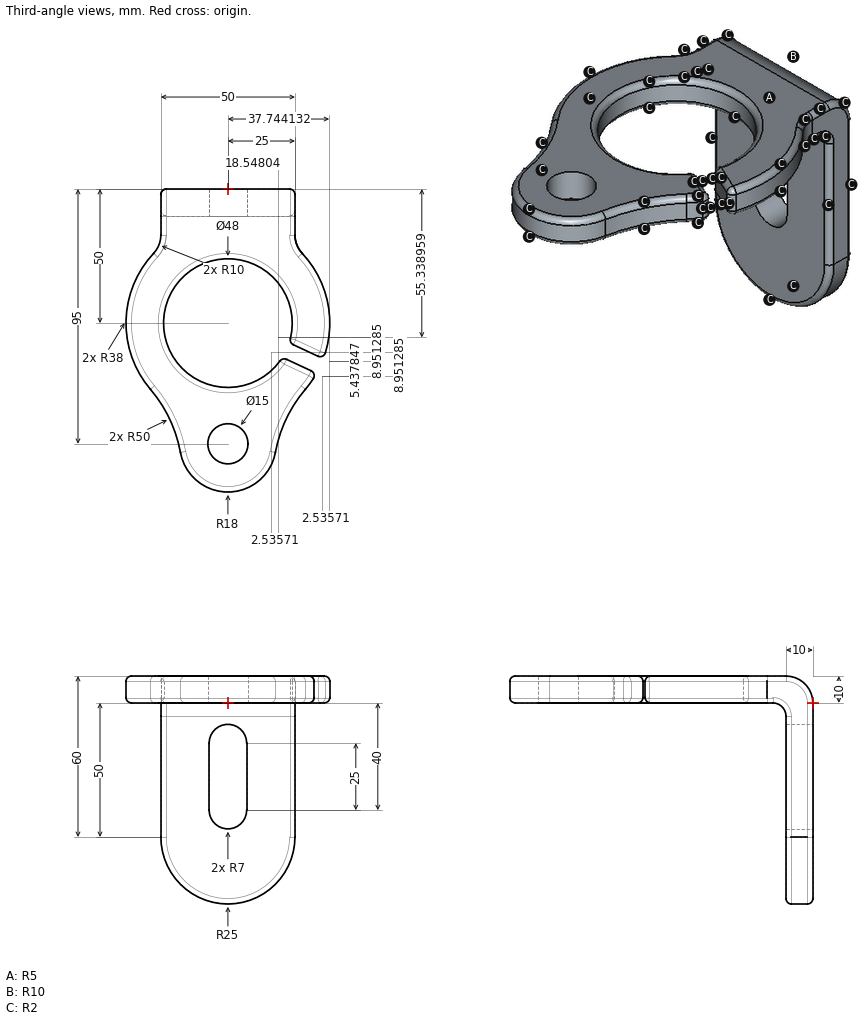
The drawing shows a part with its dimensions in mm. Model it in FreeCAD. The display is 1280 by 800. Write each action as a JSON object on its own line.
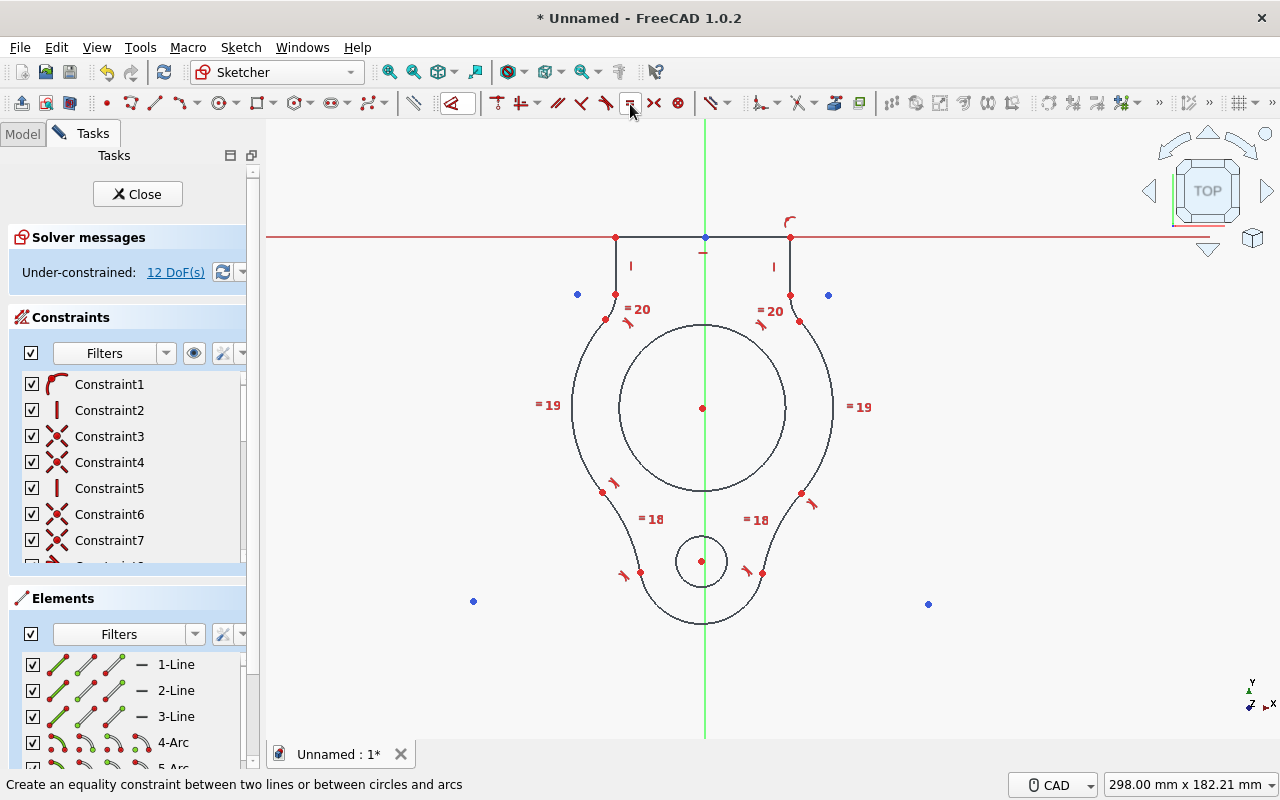
{"action": "left_click", "coordinate": [702, 408]}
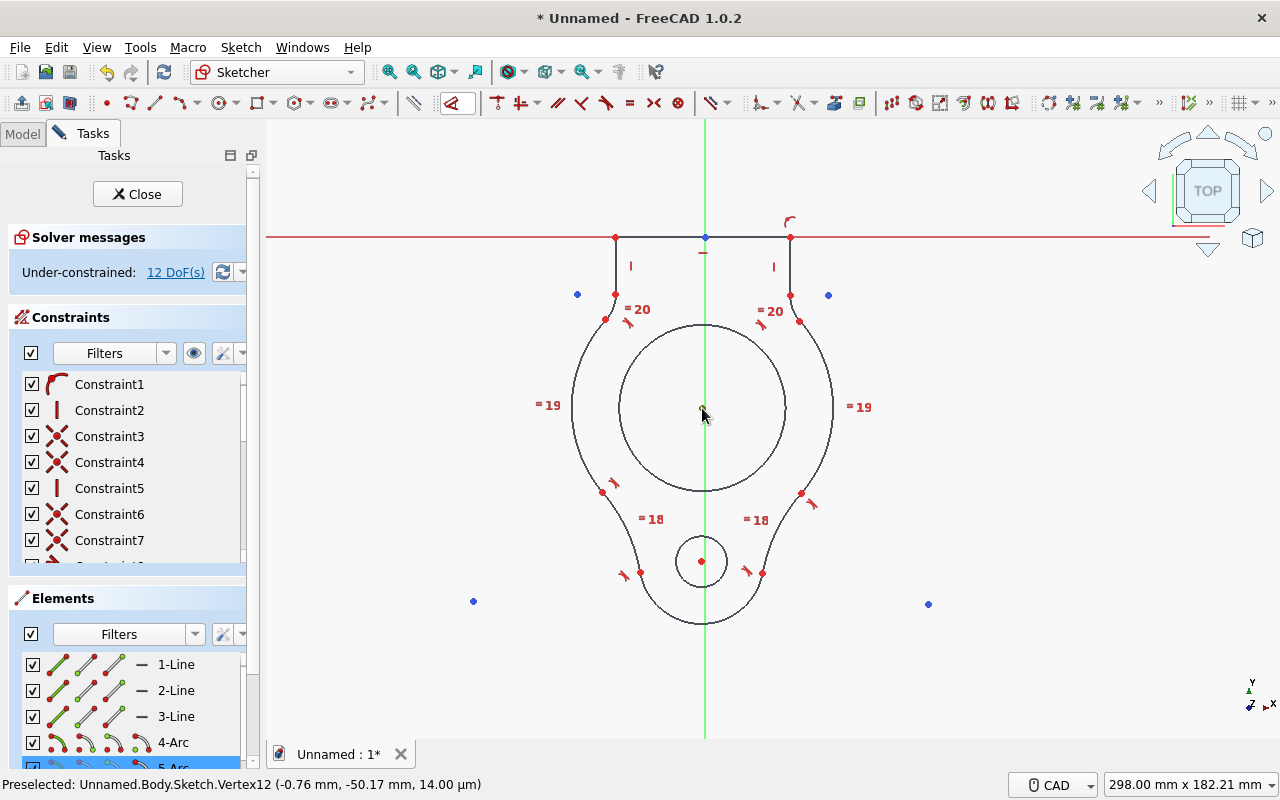
{"action": "left_click", "coordinate": [705, 671]}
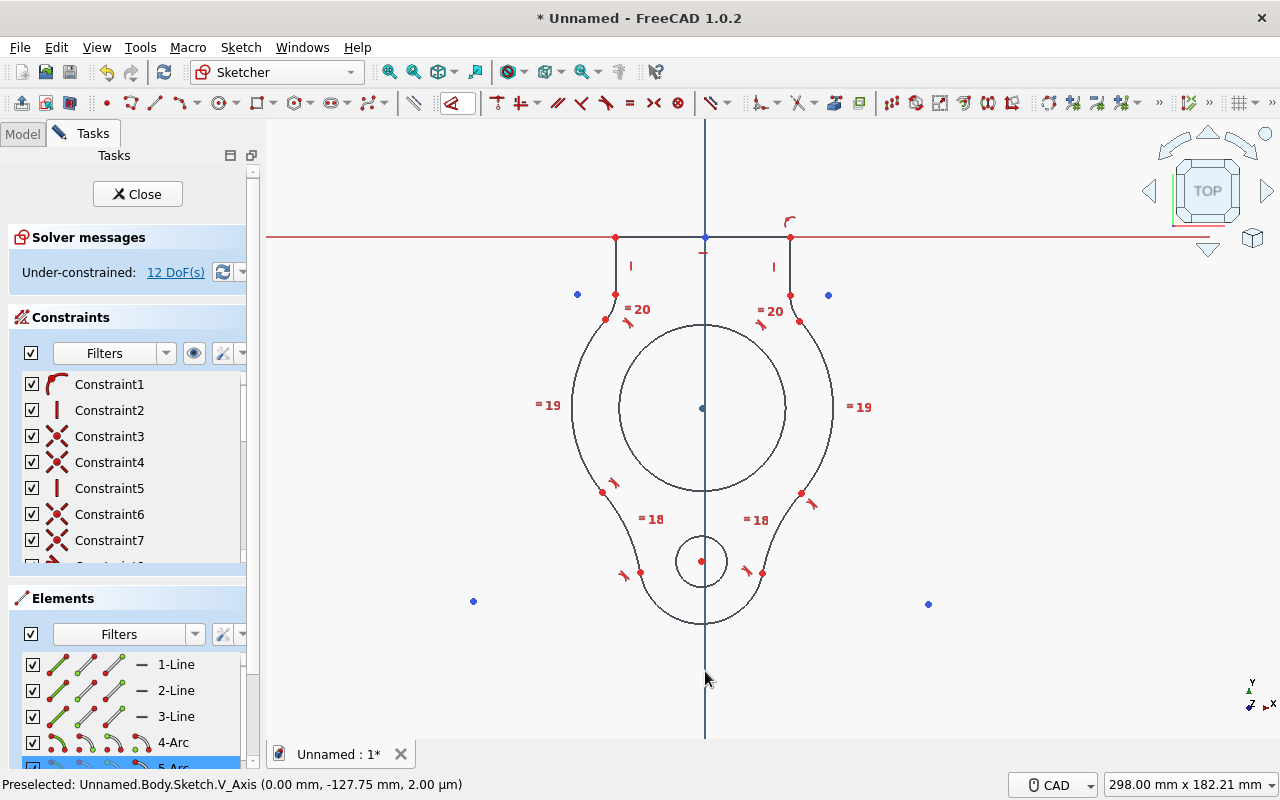
{"action": "left_click", "coordinate": [498, 104]}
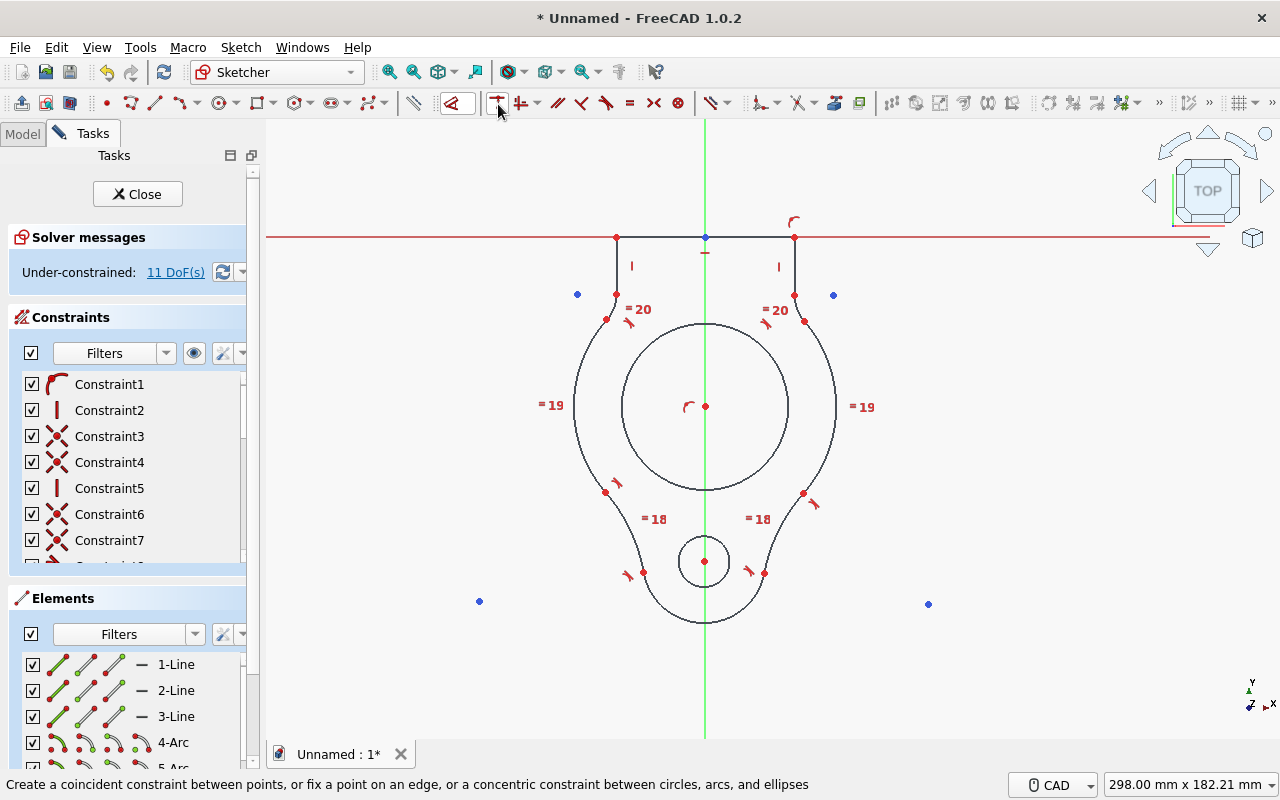
{"action": "left_click", "coordinate": [704, 562]}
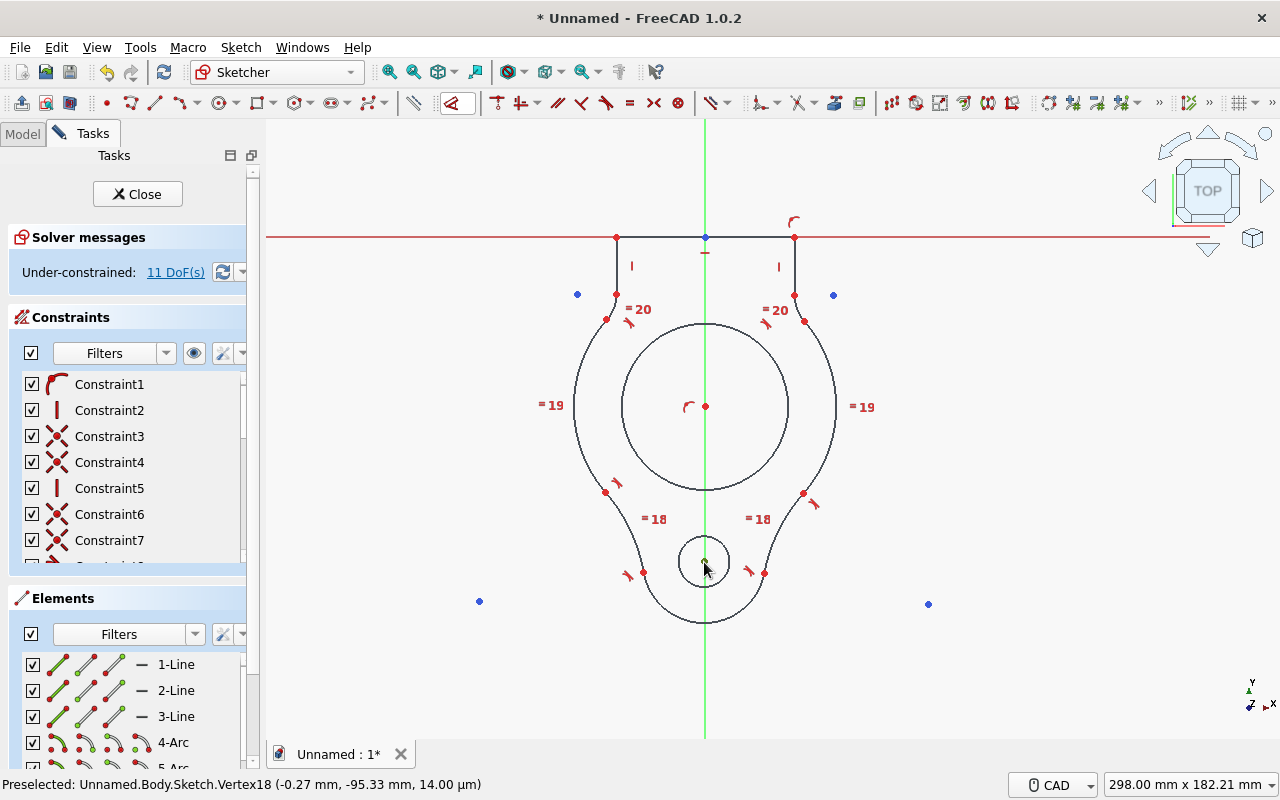
{"action": "left_click", "coordinate": [705, 671]}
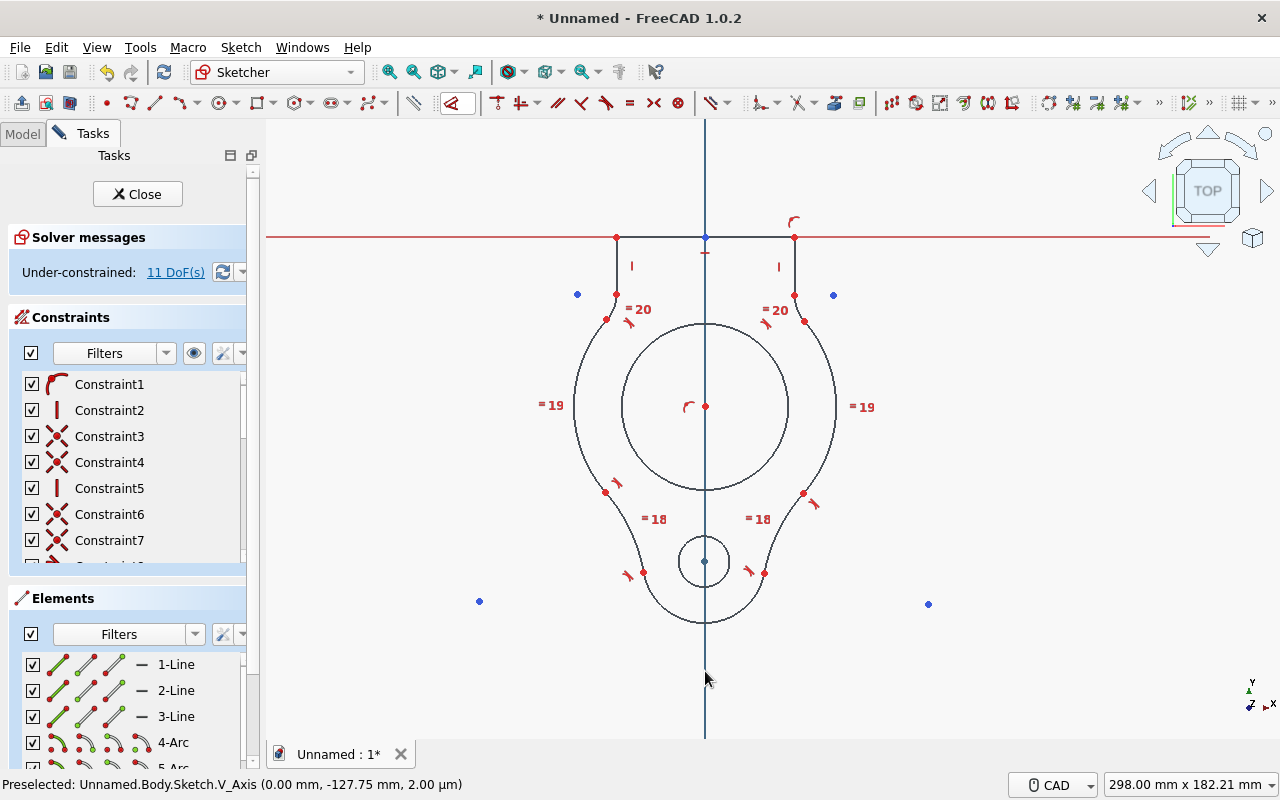
{"action": "left_click", "coordinate": [498, 104]}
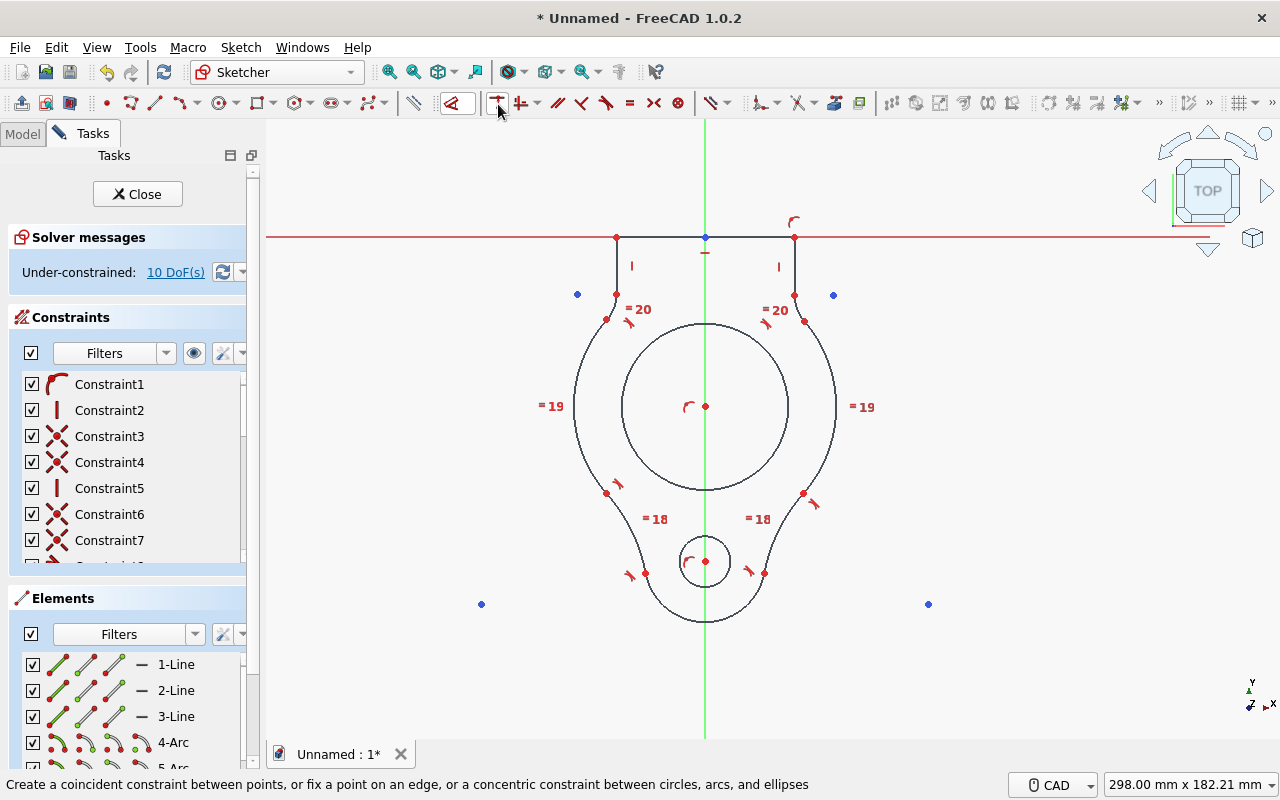
{"action": "left_click", "coordinate": [452, 104]}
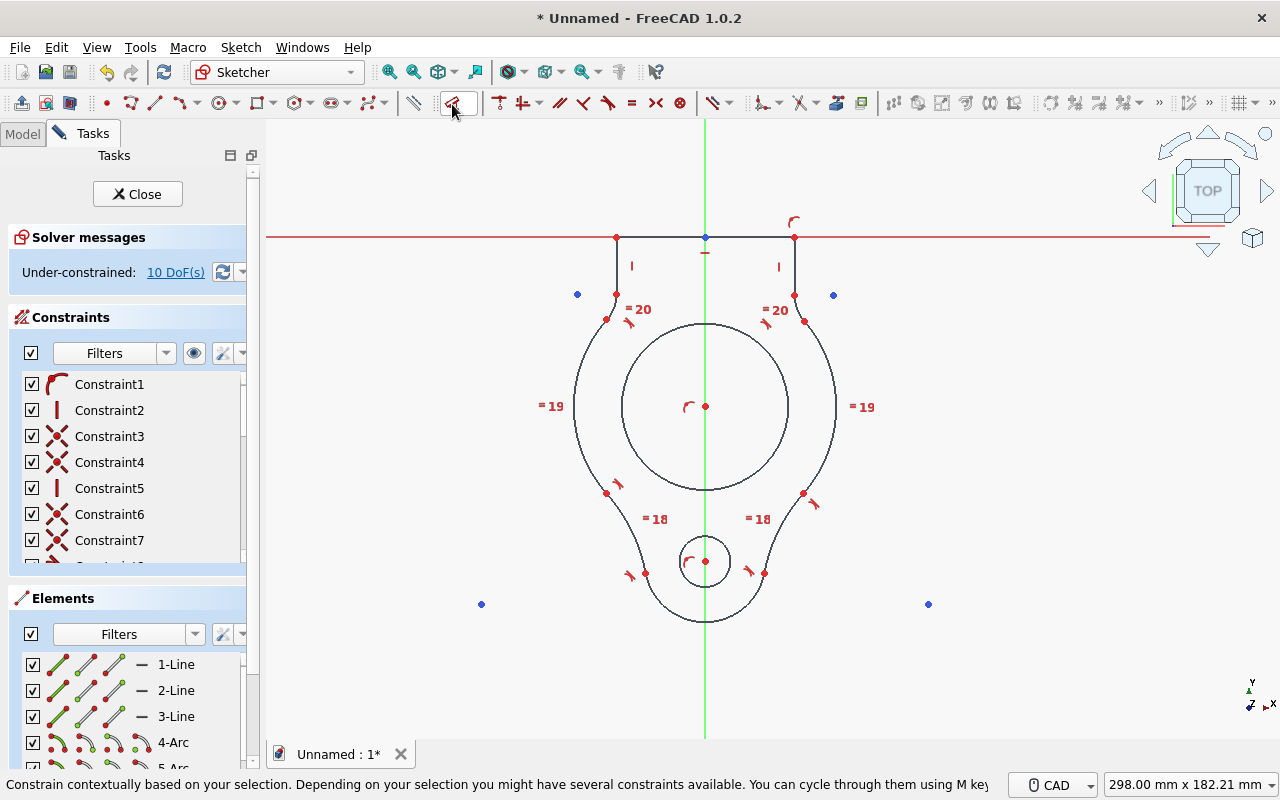
{"action": "left_click", "coordinate": [614, 308]}
{"action": "left_click", "coordinate": [644, 319]}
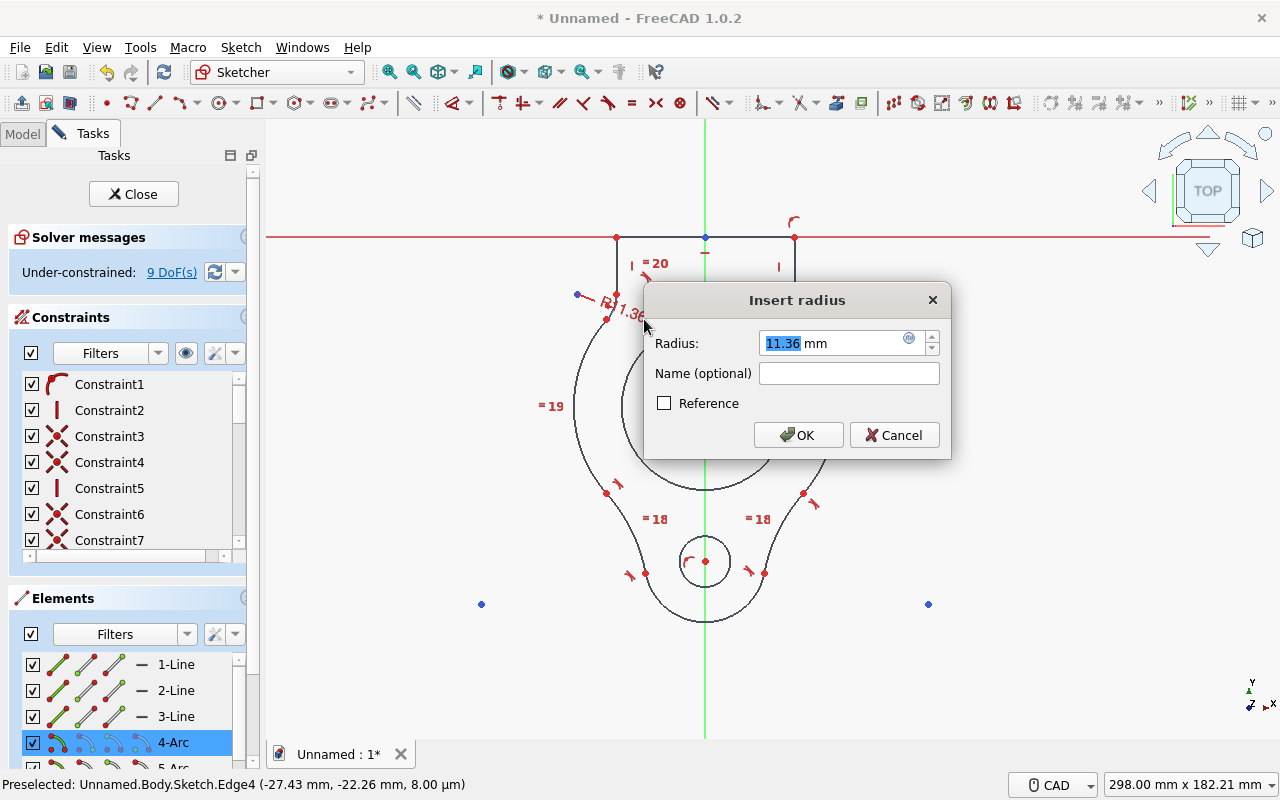
{"action": "type", "text": "10"}
{"action": "key", "text": "Return"}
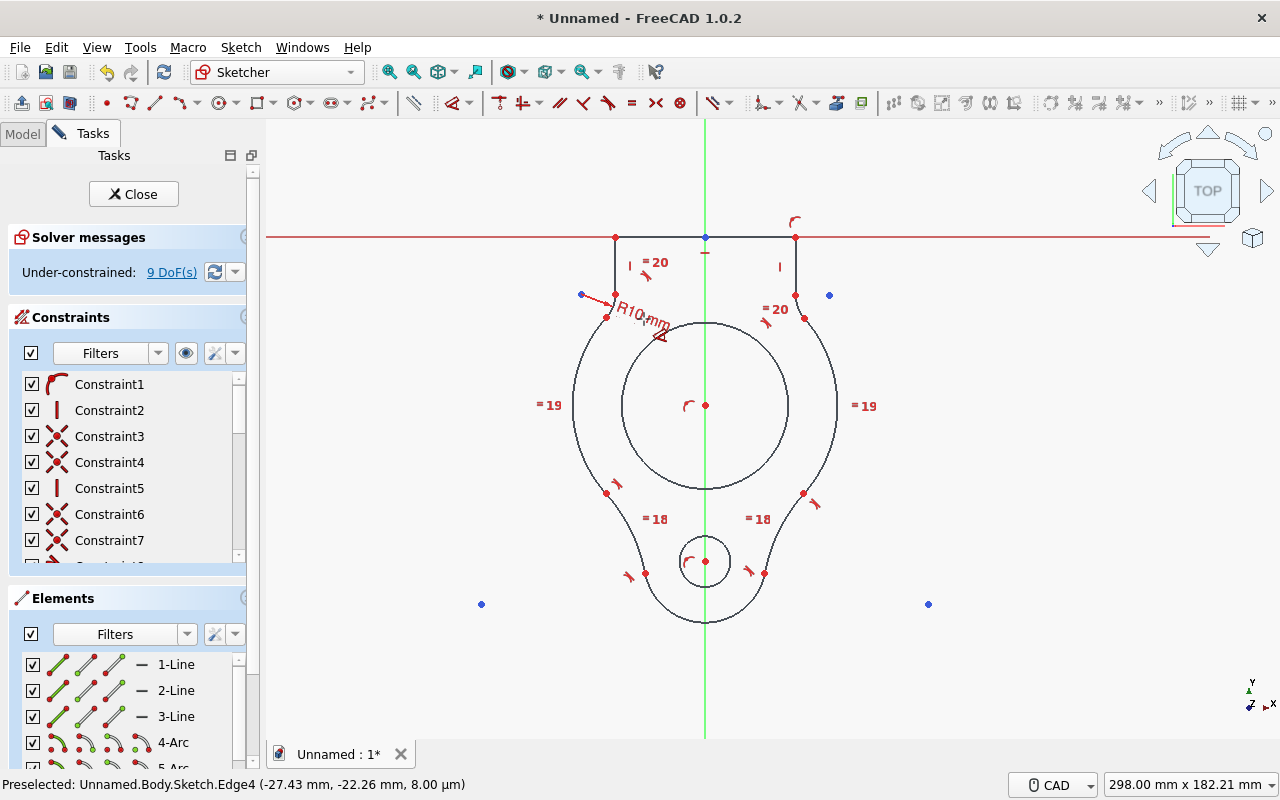
{"action": "left_click", "coordinate": [578, 367]}
{"action": "left_click", "coordinate": [547, 358]}